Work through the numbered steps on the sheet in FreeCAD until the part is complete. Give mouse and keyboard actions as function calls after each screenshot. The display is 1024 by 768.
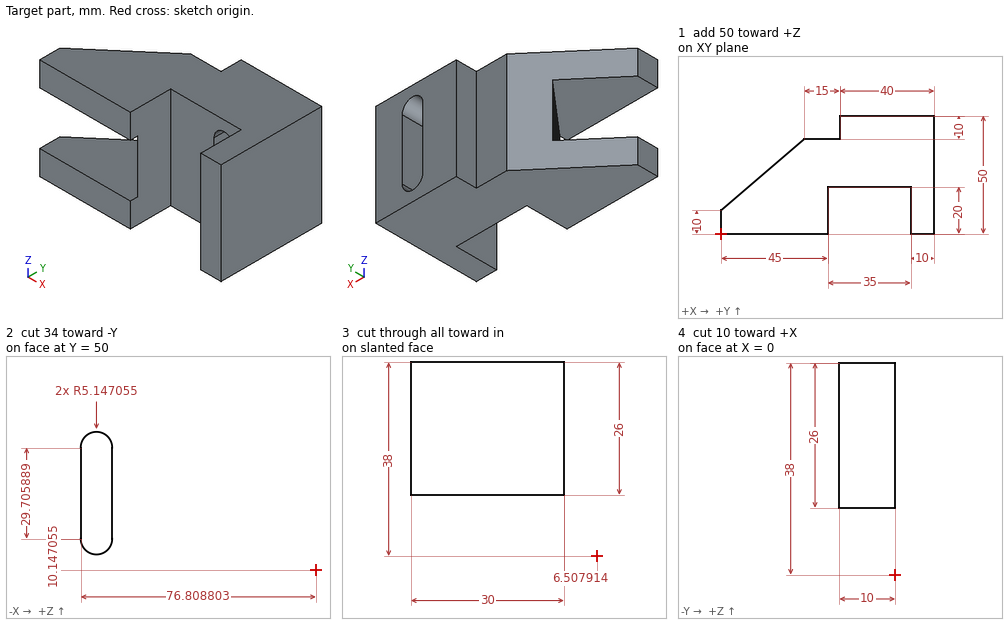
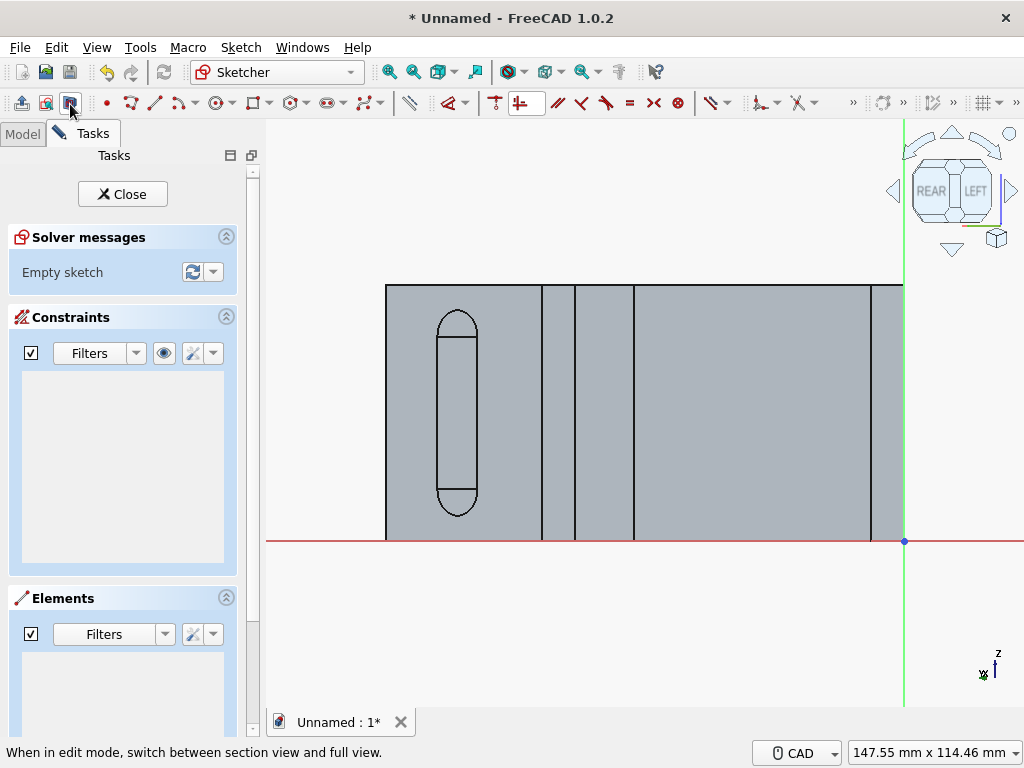
scroll(576, 413, down, 5)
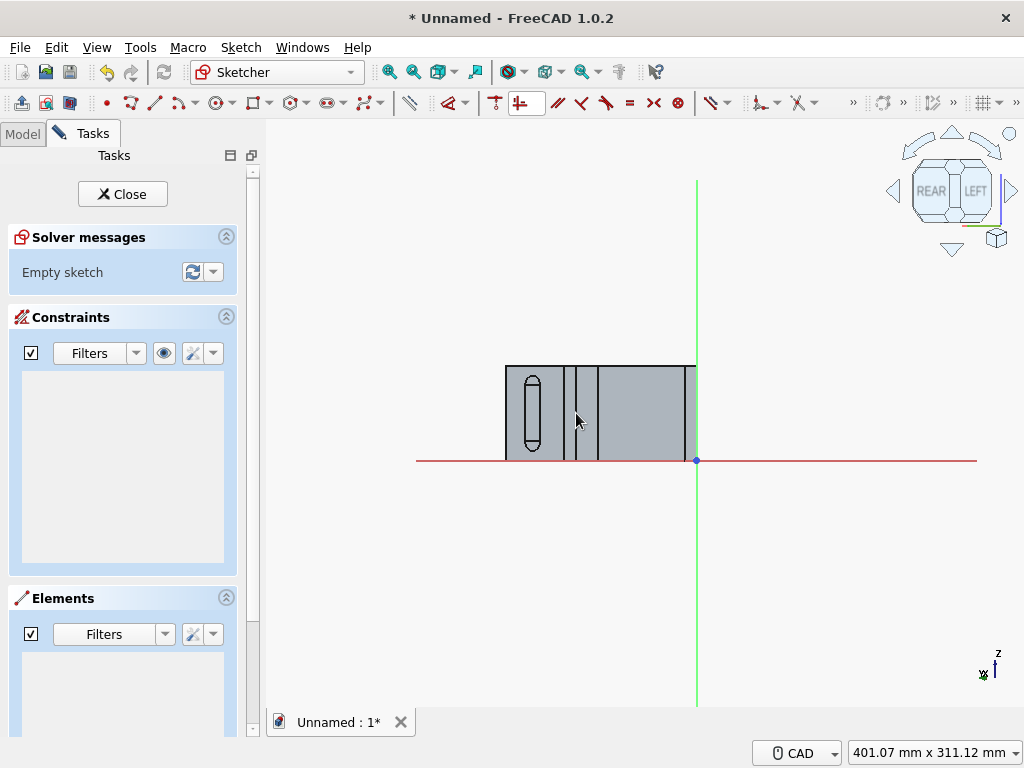
scroll(684, 428, up, 8)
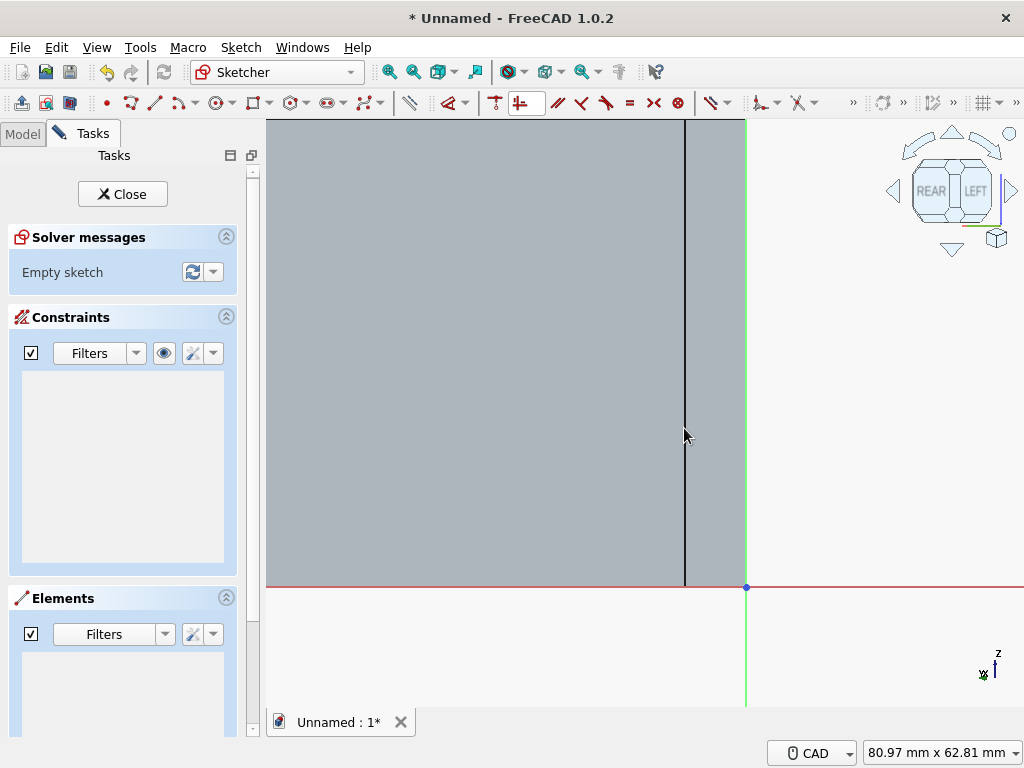
key(g)
key(r)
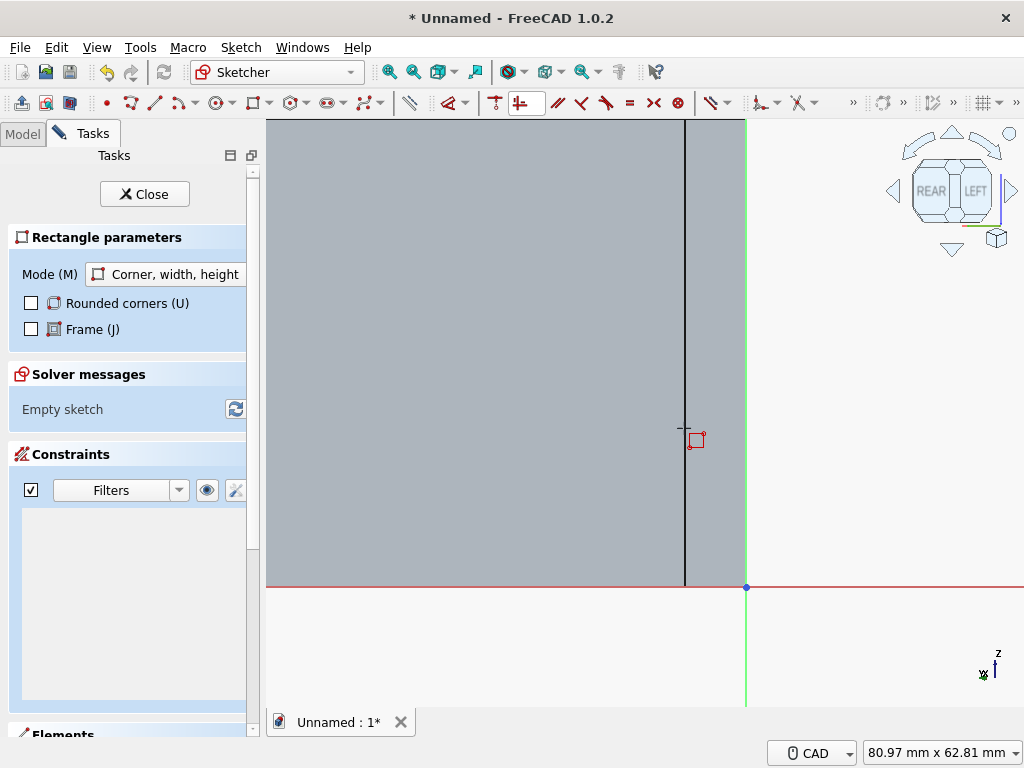
click(404, 231)
move(685, 475)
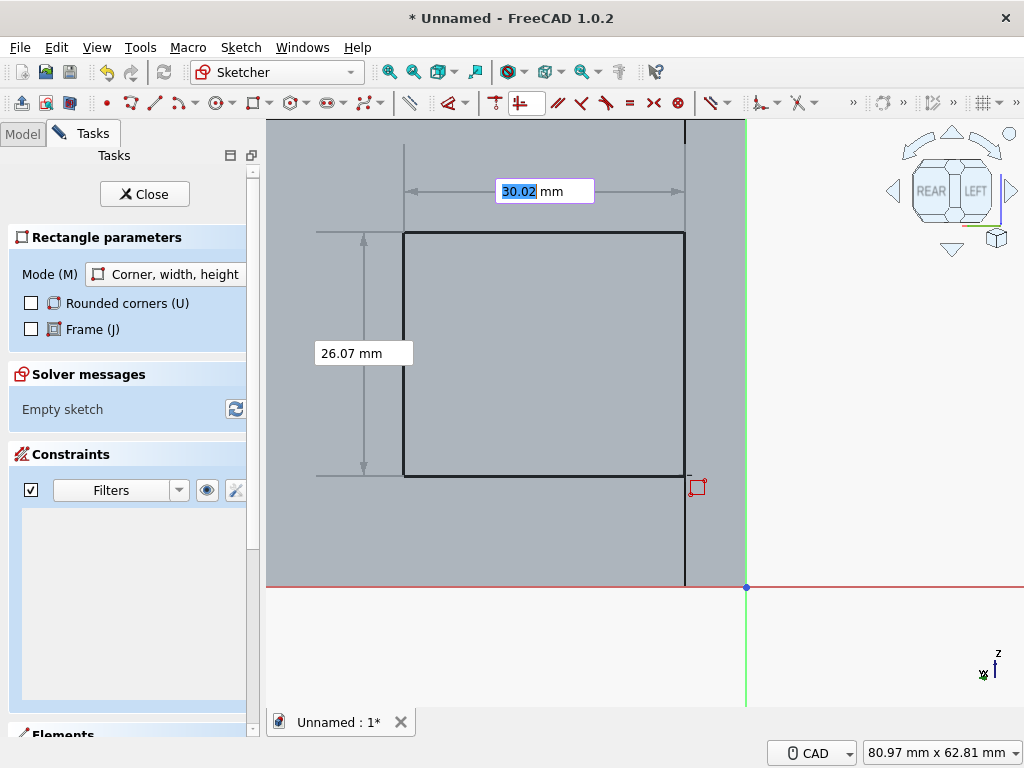
text(30)
key(Tab)
text(26)
key(Return)
key(Escape)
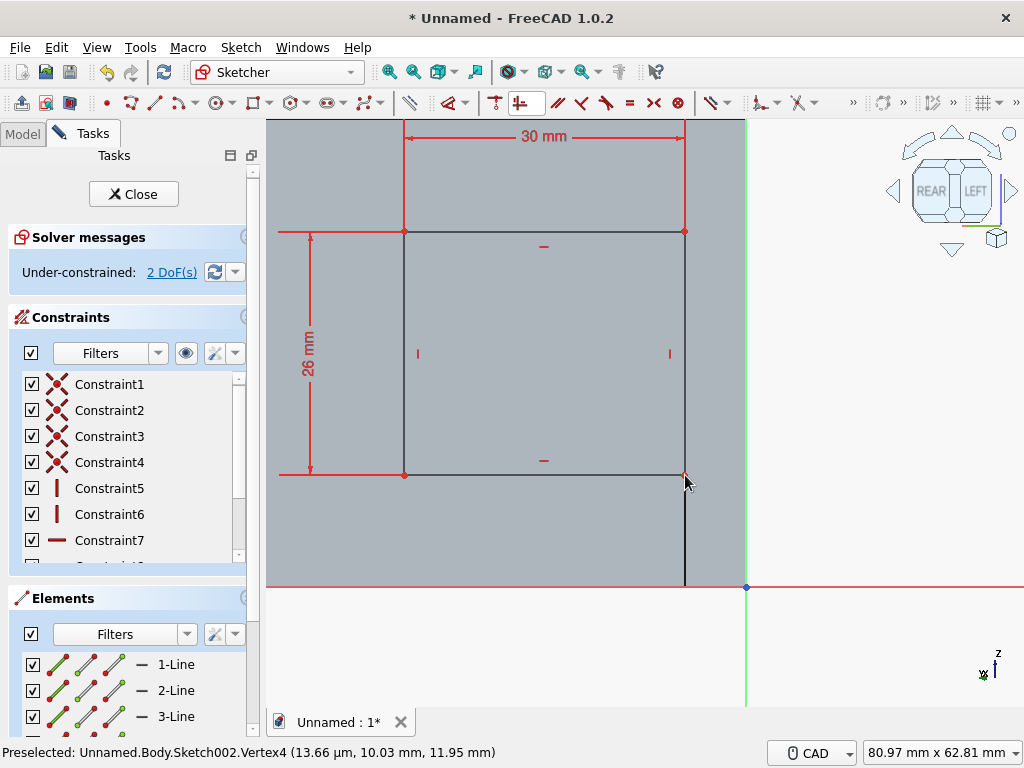
click(448, 104)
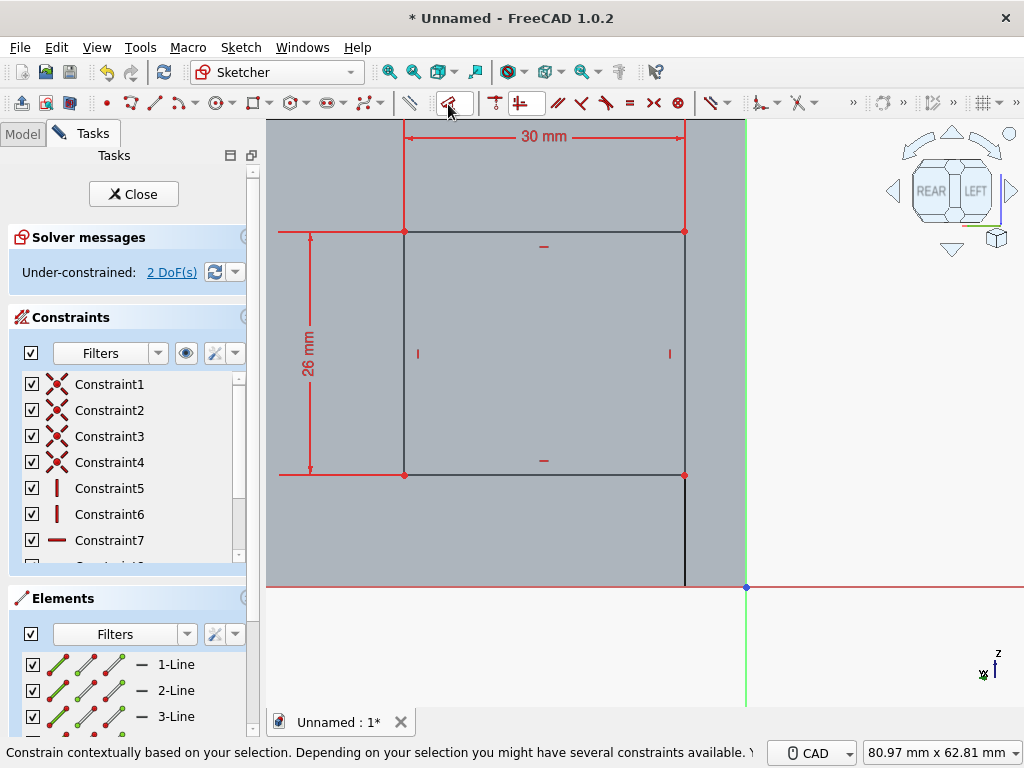
click(404, 232)
click(370, 410)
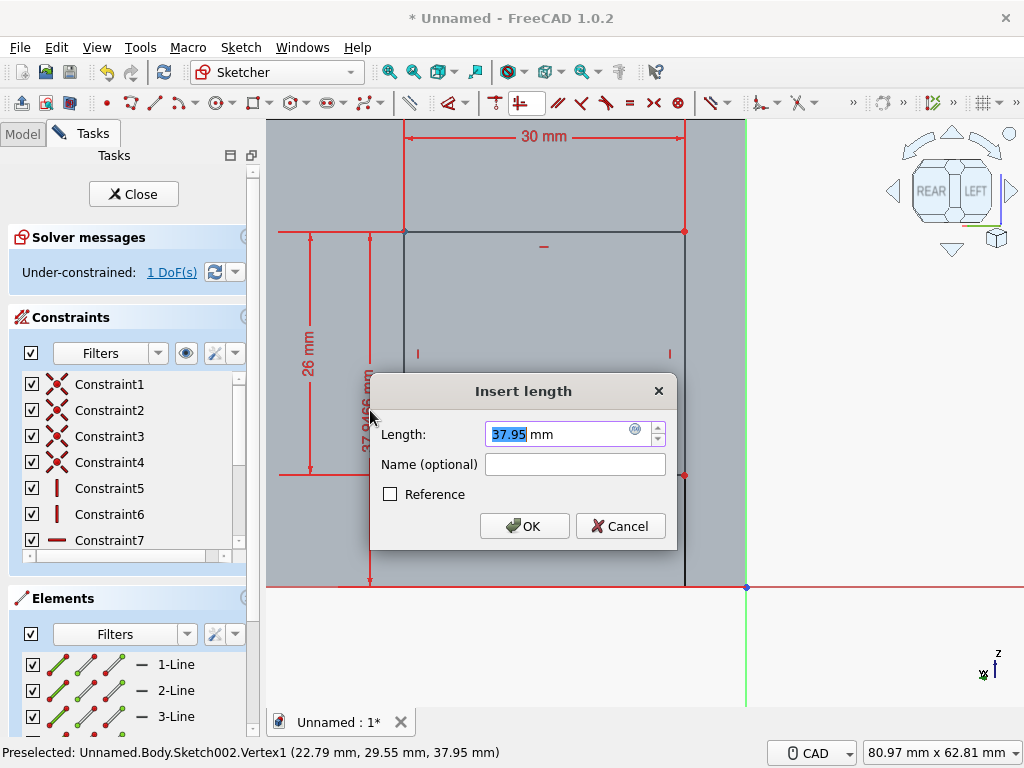
text(38)
key(Return)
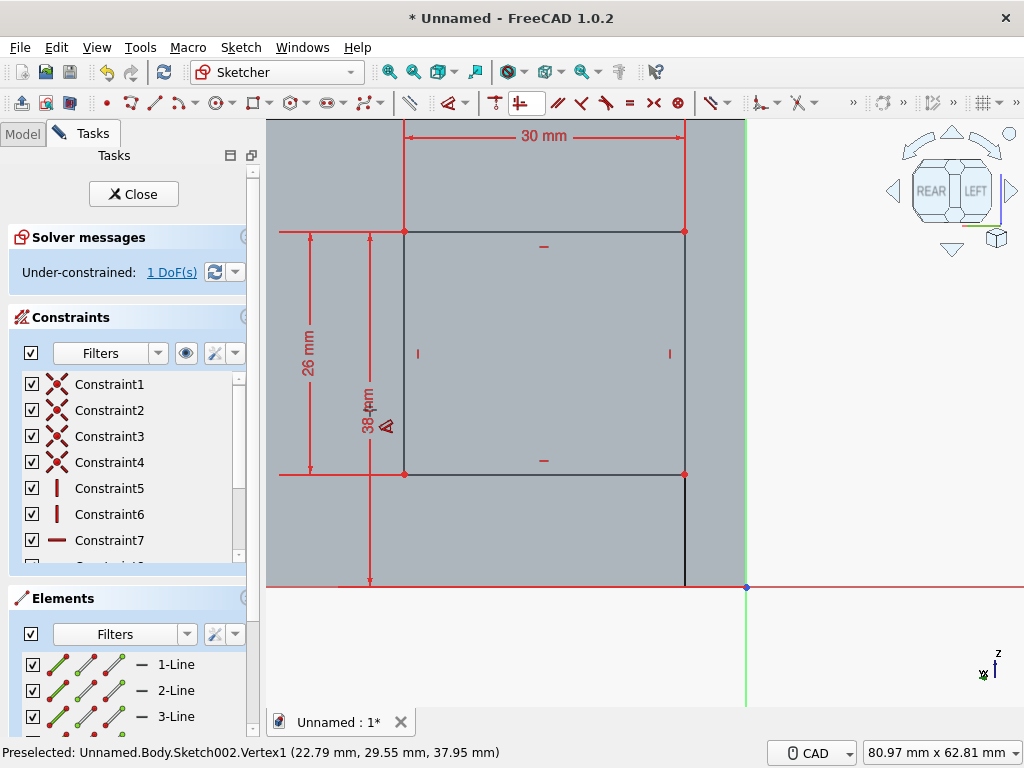
click(685, 475)
click(715, 621)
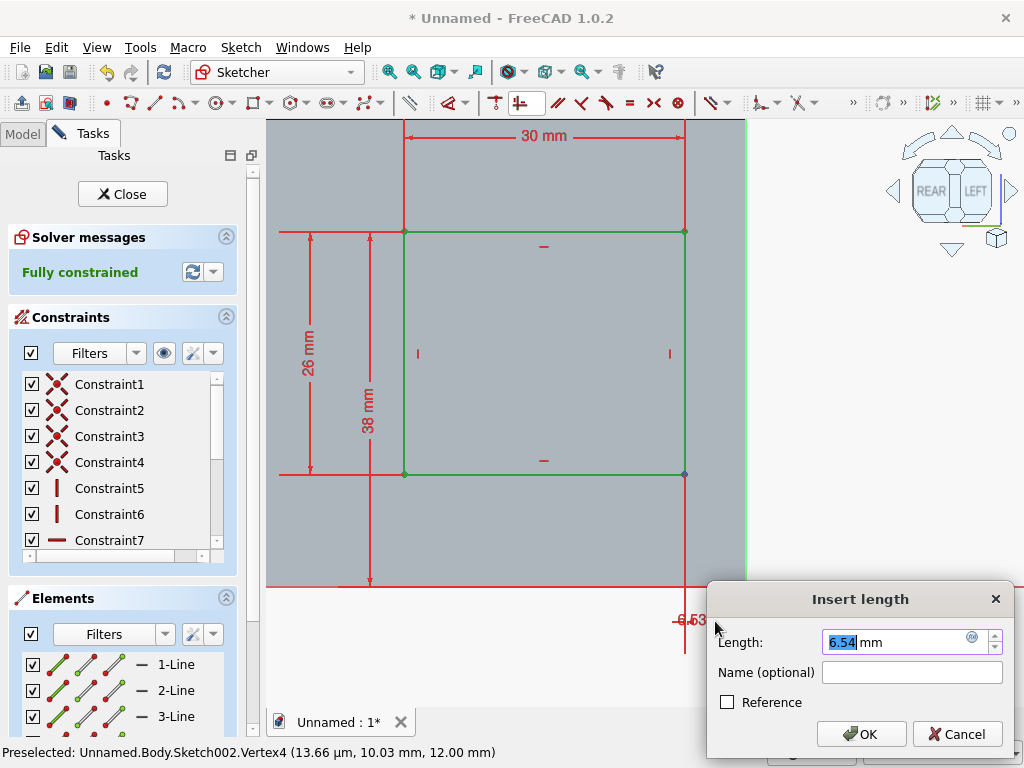
text(6.507914)
key(Return)
key(Escape)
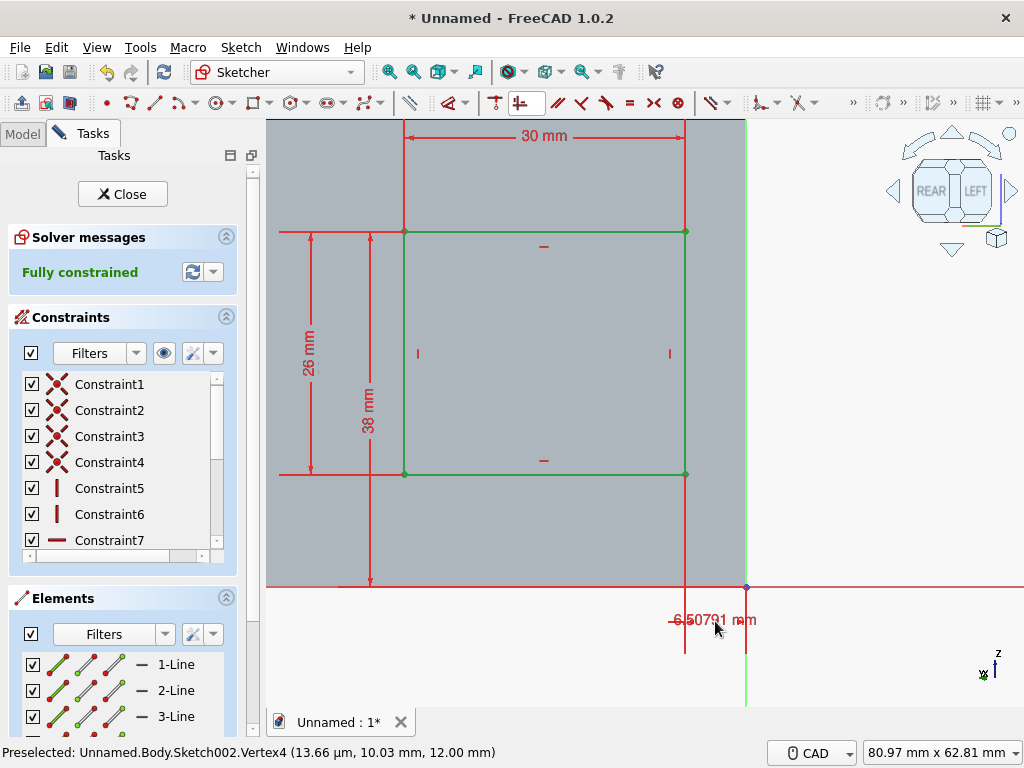
click(123, 194)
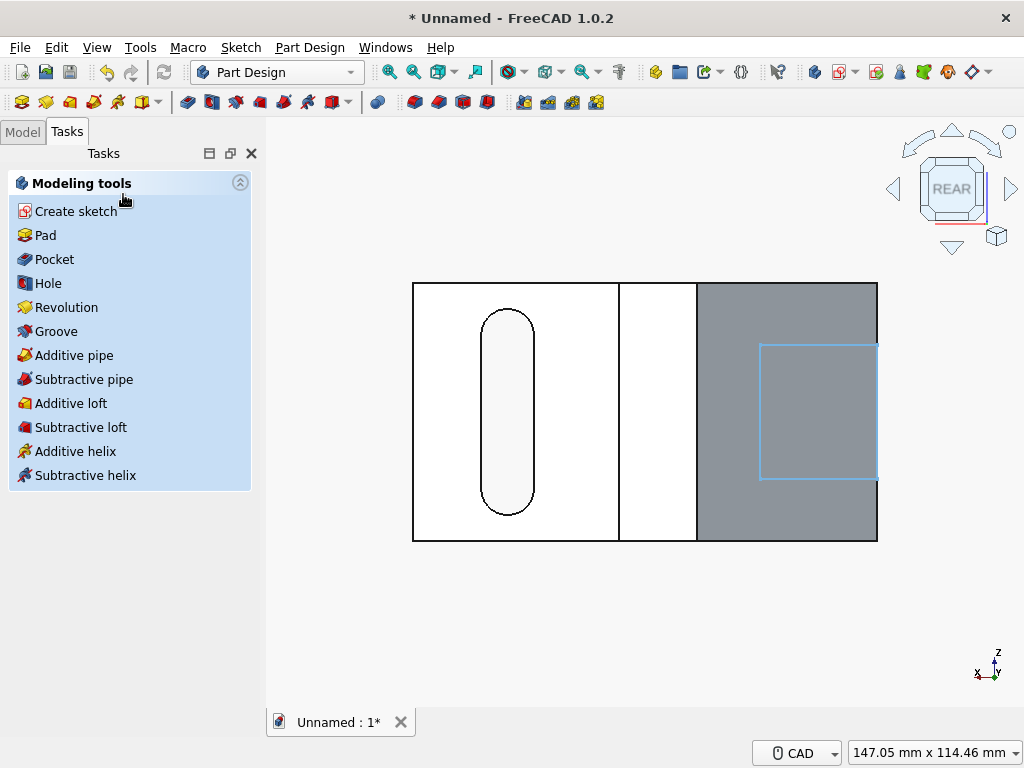
click(188, 102)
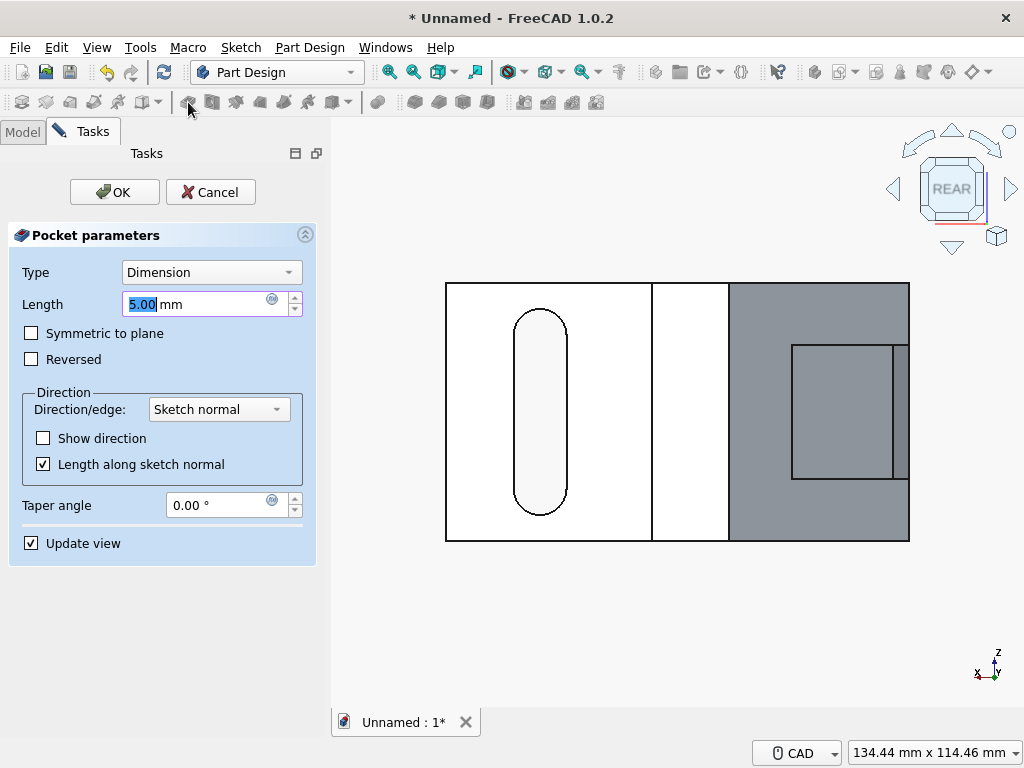
click(212, 272)